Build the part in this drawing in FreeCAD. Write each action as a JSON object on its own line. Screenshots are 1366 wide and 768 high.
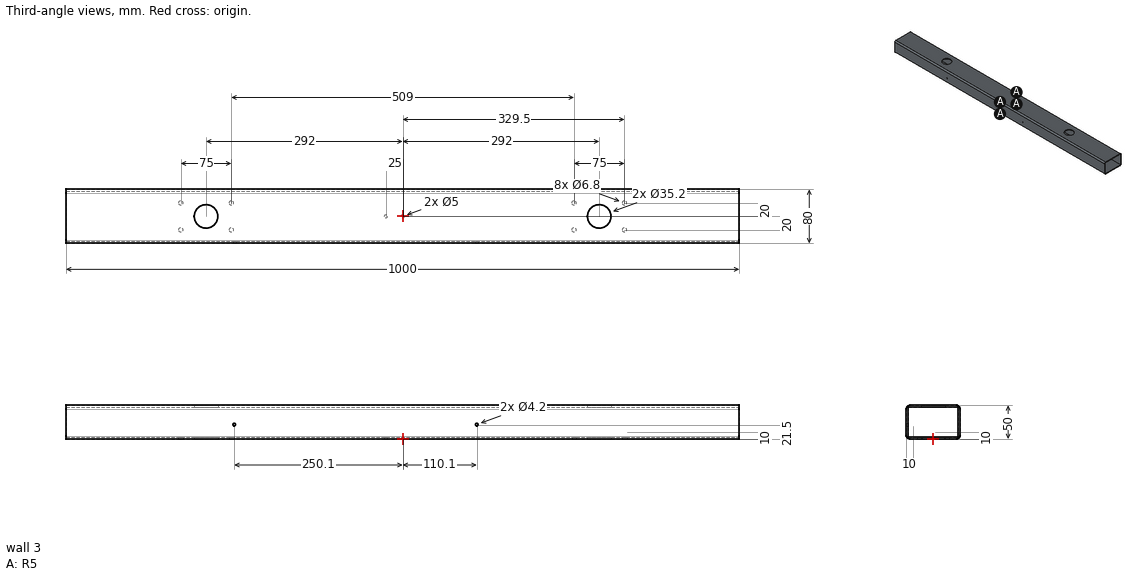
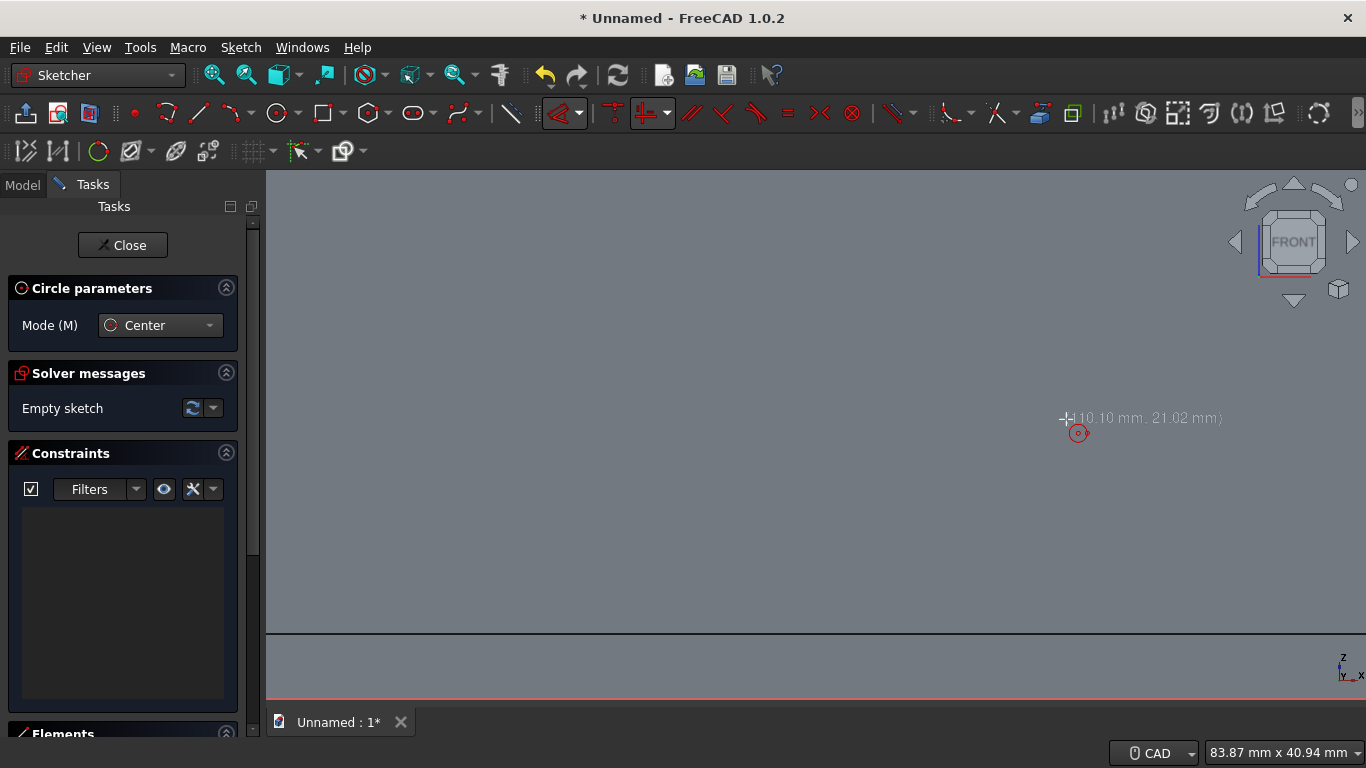
{"action": "scroll", "coordinate": [1068, 422], "scroll_direction": "down", "scroll_amount": 10}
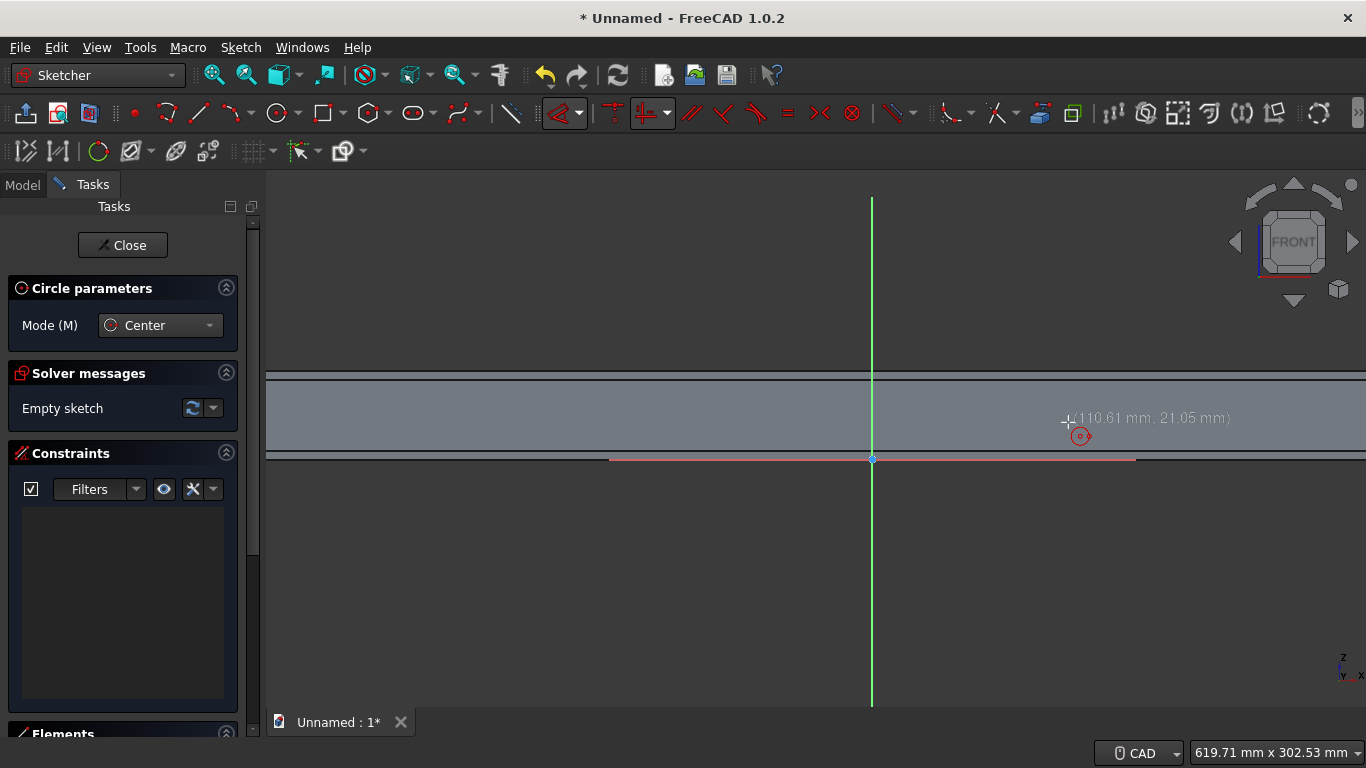
{"action": "left_click", "coordinate": [1068, 422]}
{"action": "mouse_move", "coordinate": [1070, 419]}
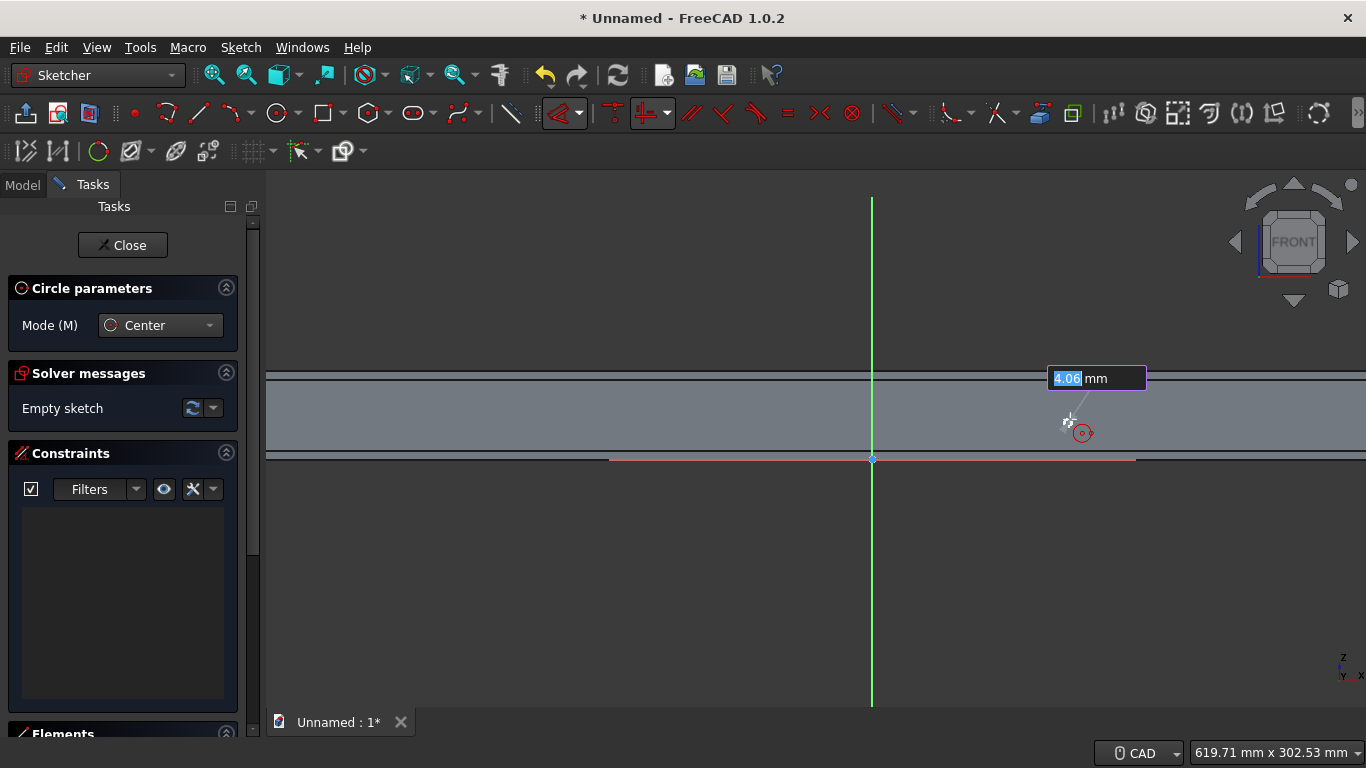
{"action": "type", "text": "4.2"}
{"action": "key", "text": "Return"}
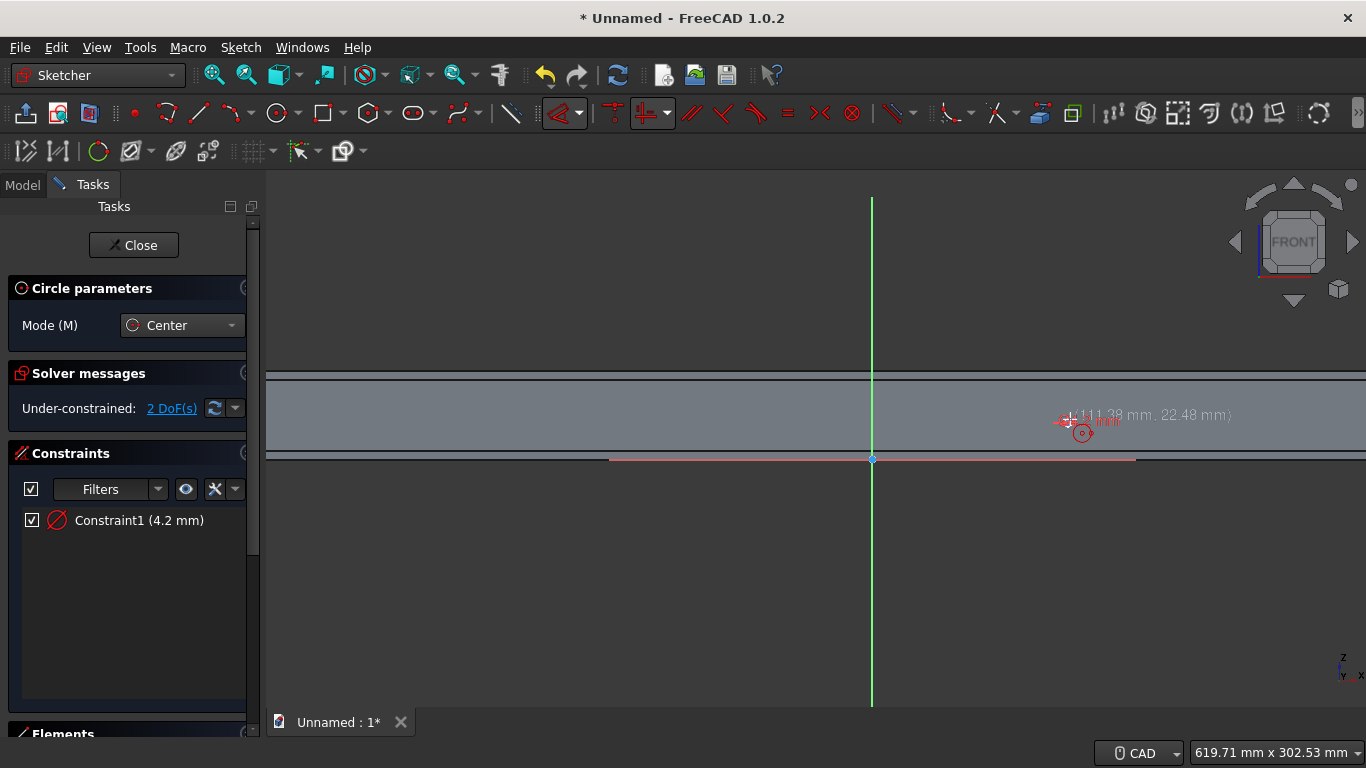
{"action": "scroll", "coordinate": [428, 422], "scroll_direction": "up", "scroll_amount": 10}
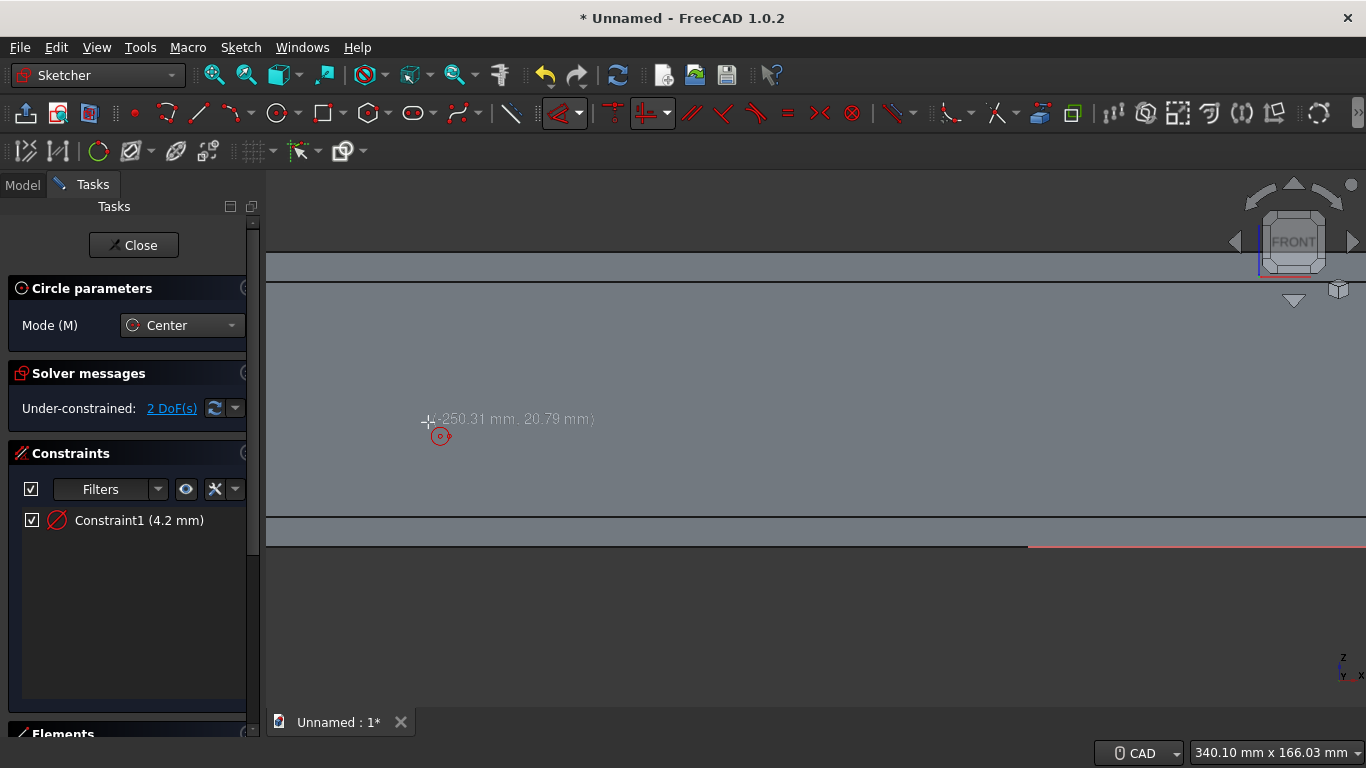
{"action": "scroll", "coordinate": [428, 422], "scroll_direction": "down", "scroll_amount": 10}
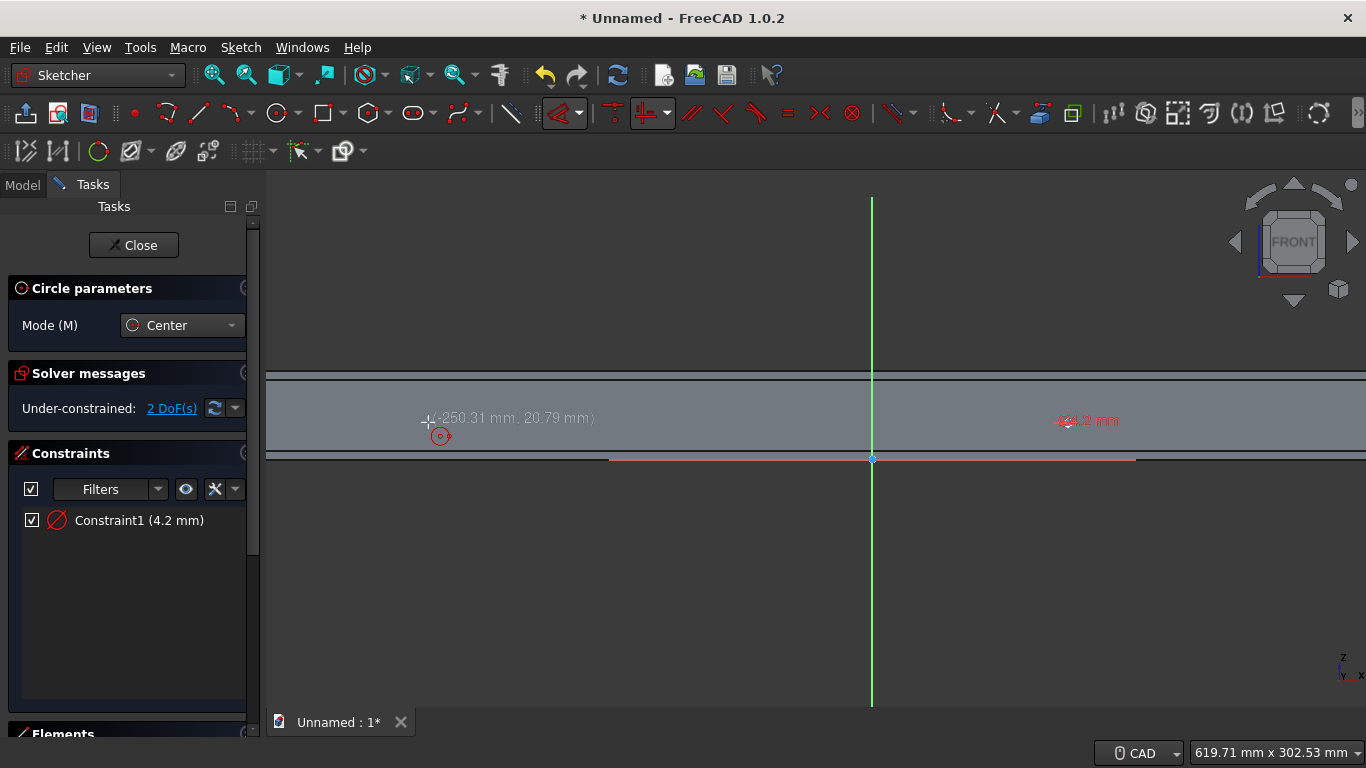
{"action": "left_click", "coordinate": [428, 422]}
{"action": "mouse_move", "coordinate": [431, 419]}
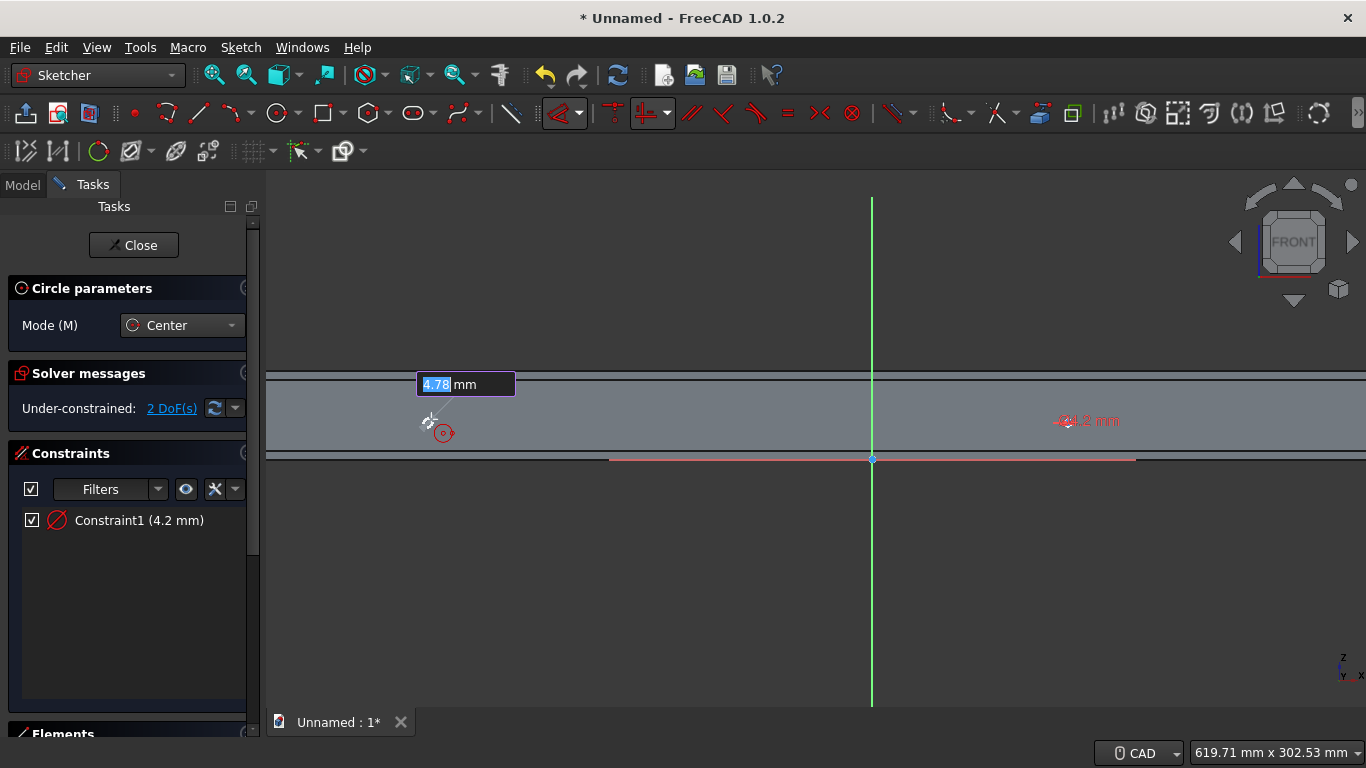
{"action": "type", "text": "4.2"}
{"action": "key", "text": "Return"}
{"action": "key", "text": "Escape"}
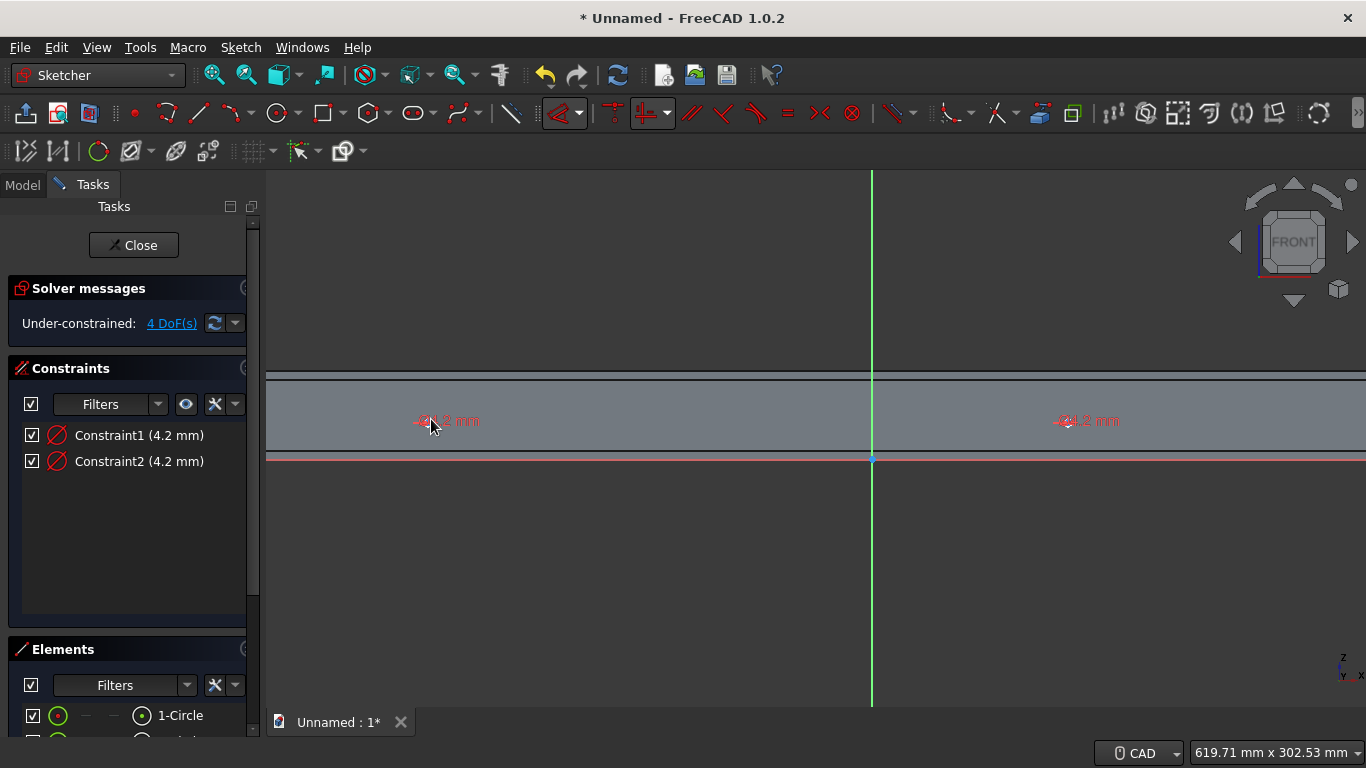
{"action": "left_click", "coordinate": [1068, 423]}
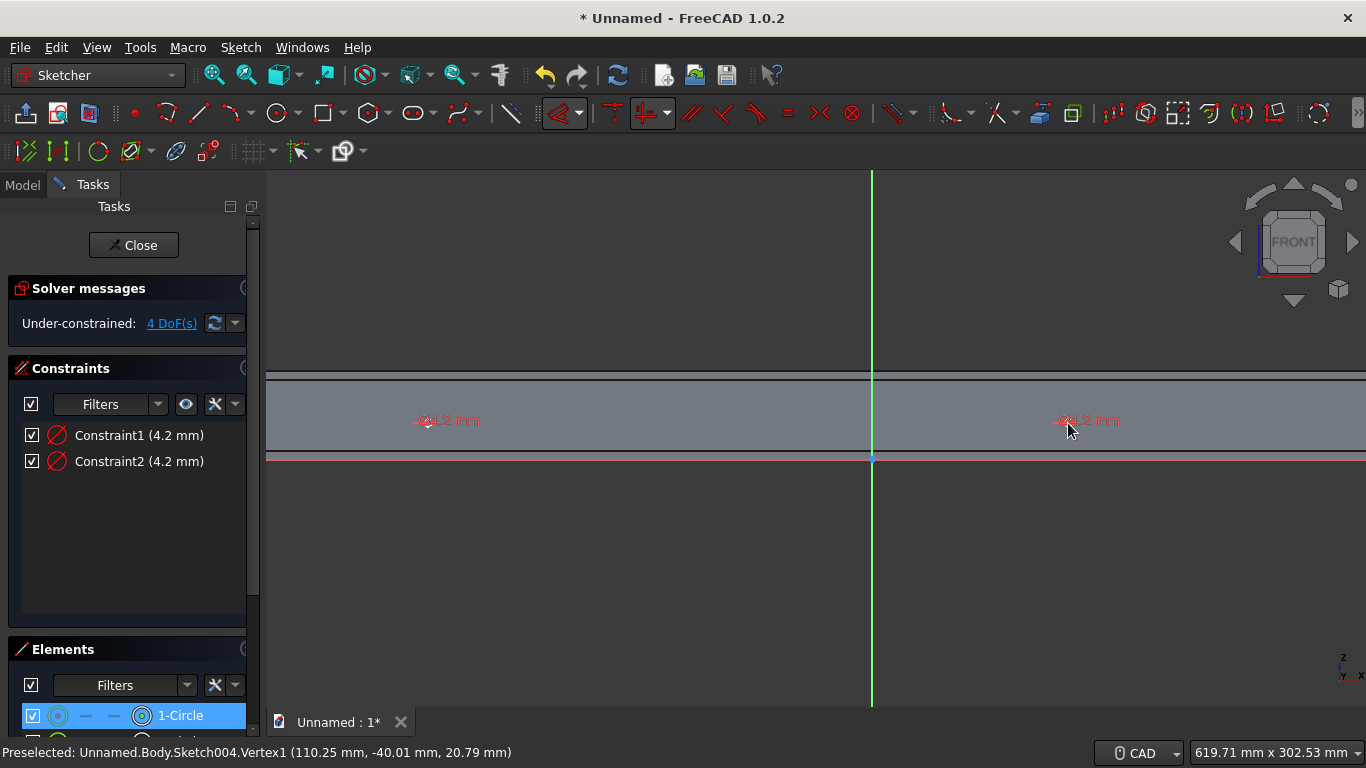
{"action": "left_click", "coordinate": [428, 423]}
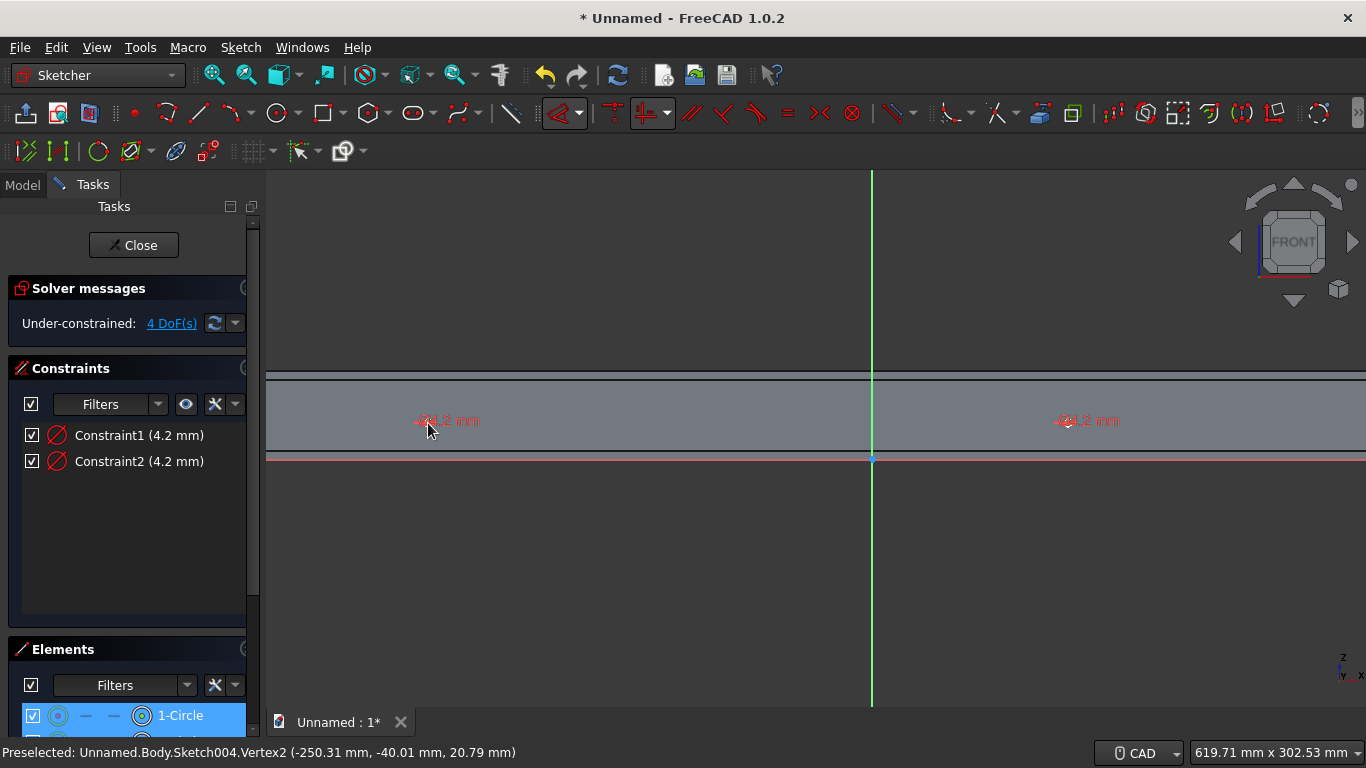
{"action": "key", "text": "h"}